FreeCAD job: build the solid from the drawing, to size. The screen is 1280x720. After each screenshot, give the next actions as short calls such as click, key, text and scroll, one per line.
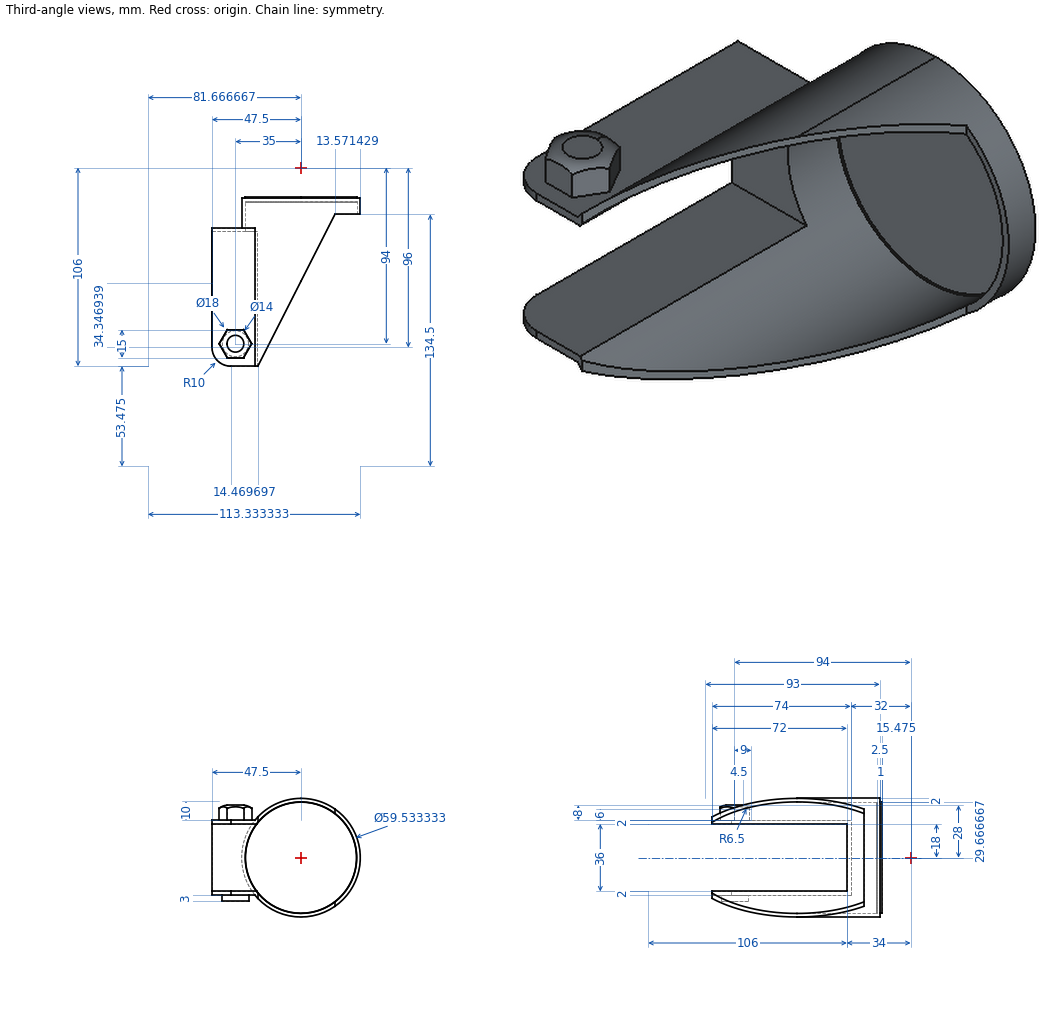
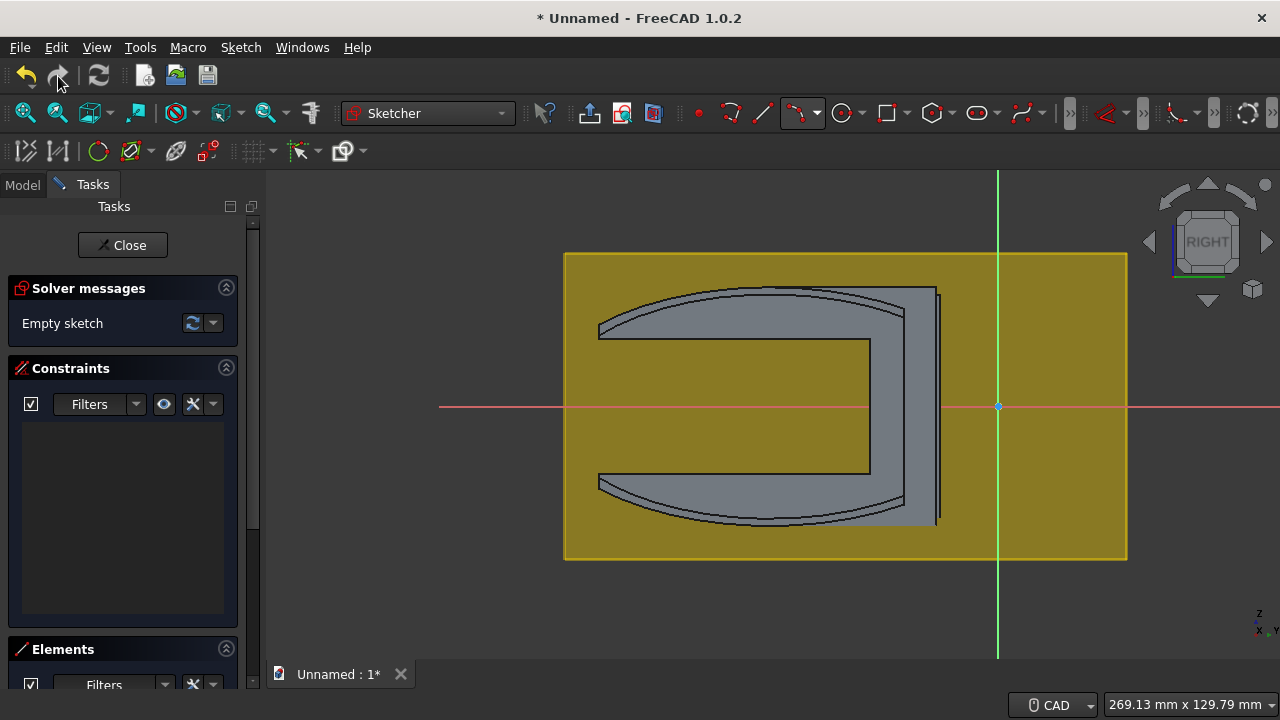
click(654, 114)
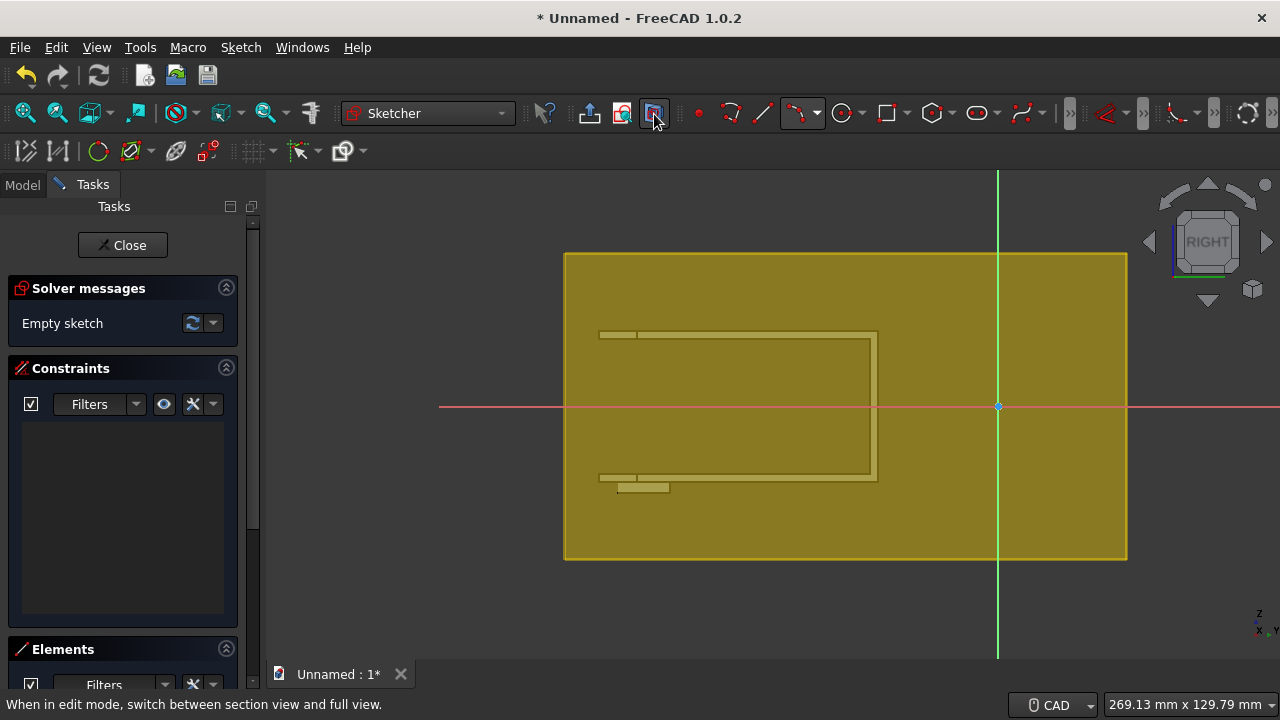
scroll(654, 294, up, 10)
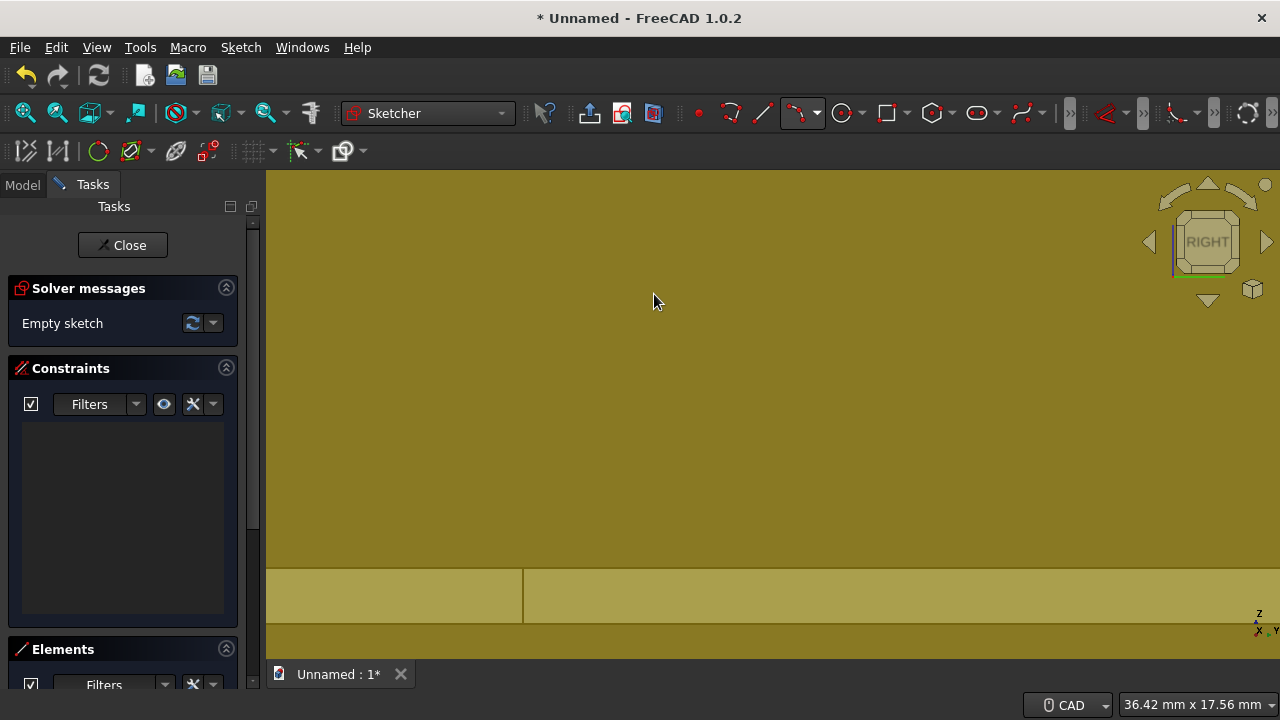
key(g)
key(m)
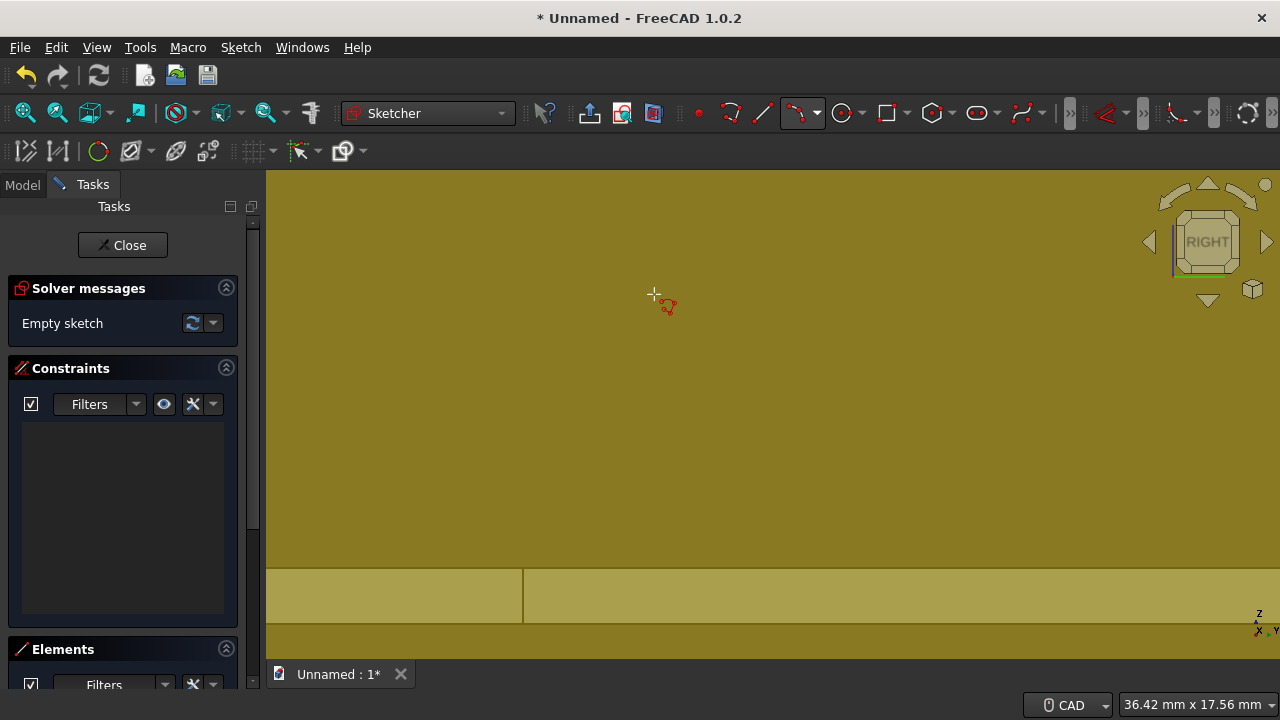
click(704, 345)
click(578, 345)
click(578, 568)
click(829, 568)
click(829, 401)
right_click(829, 401)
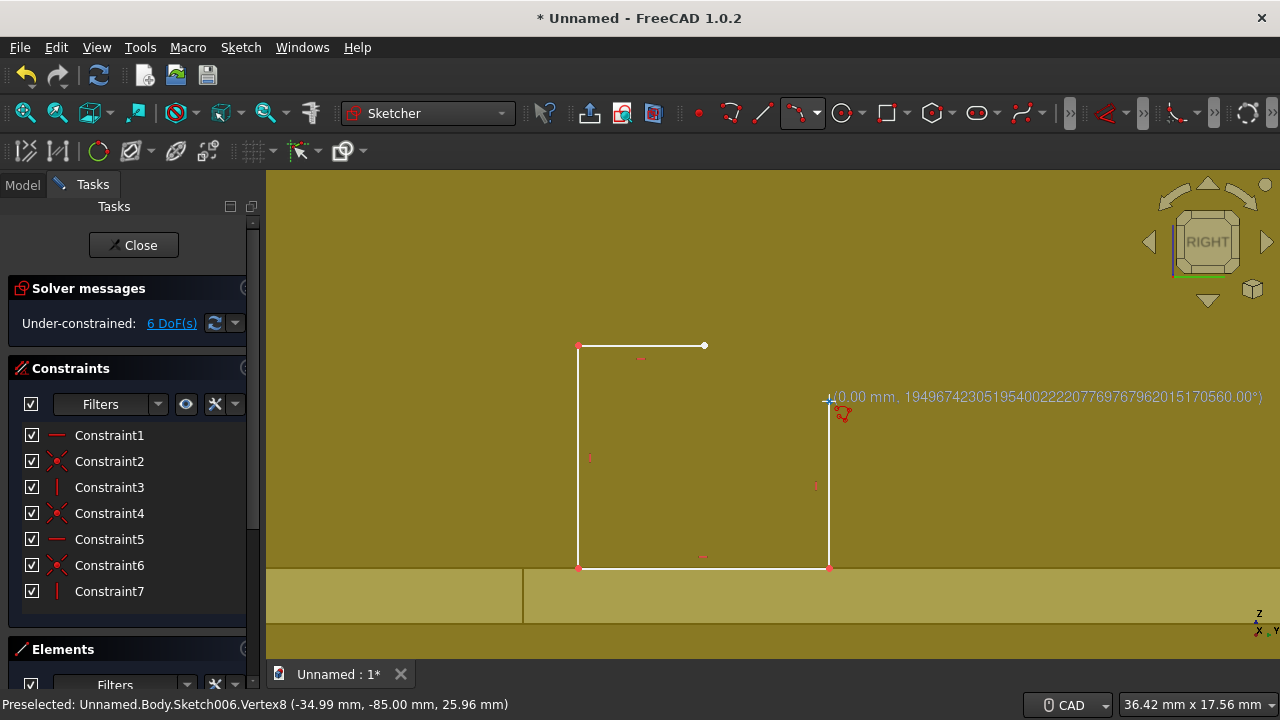
key(g)
key(3)
key(a)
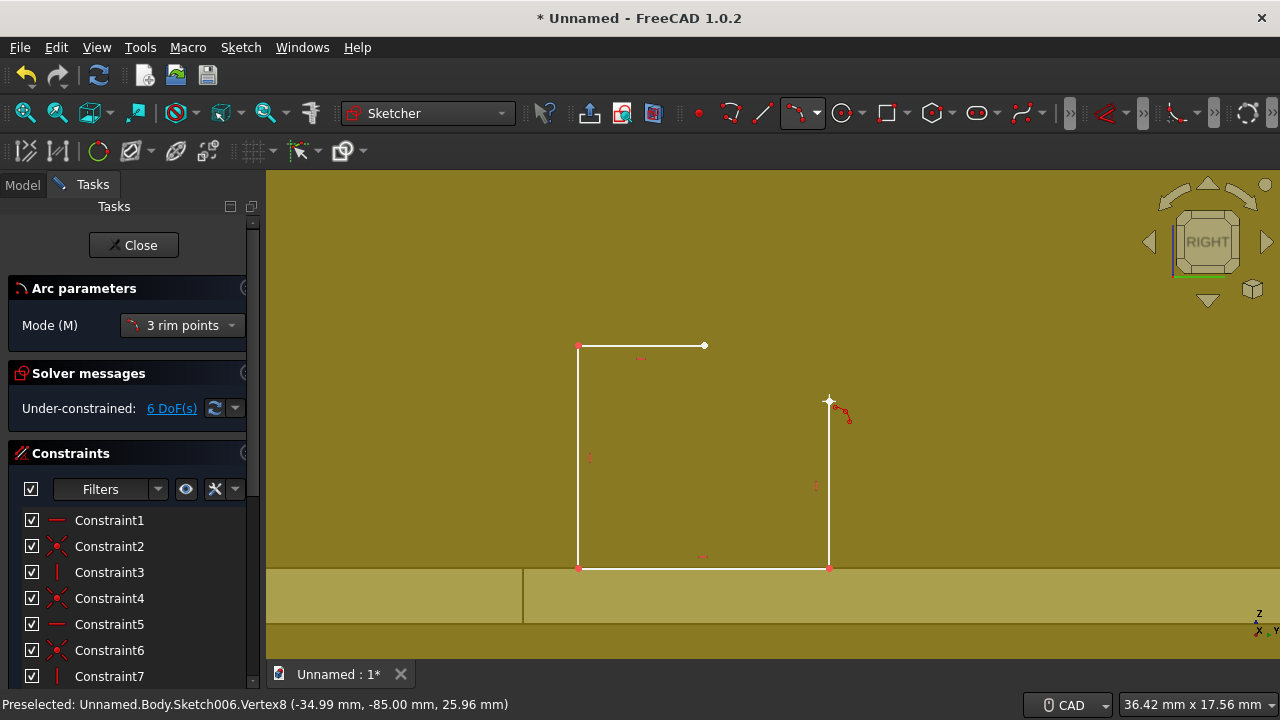
click(829, 402)
click(704, 346)
click(772, 361)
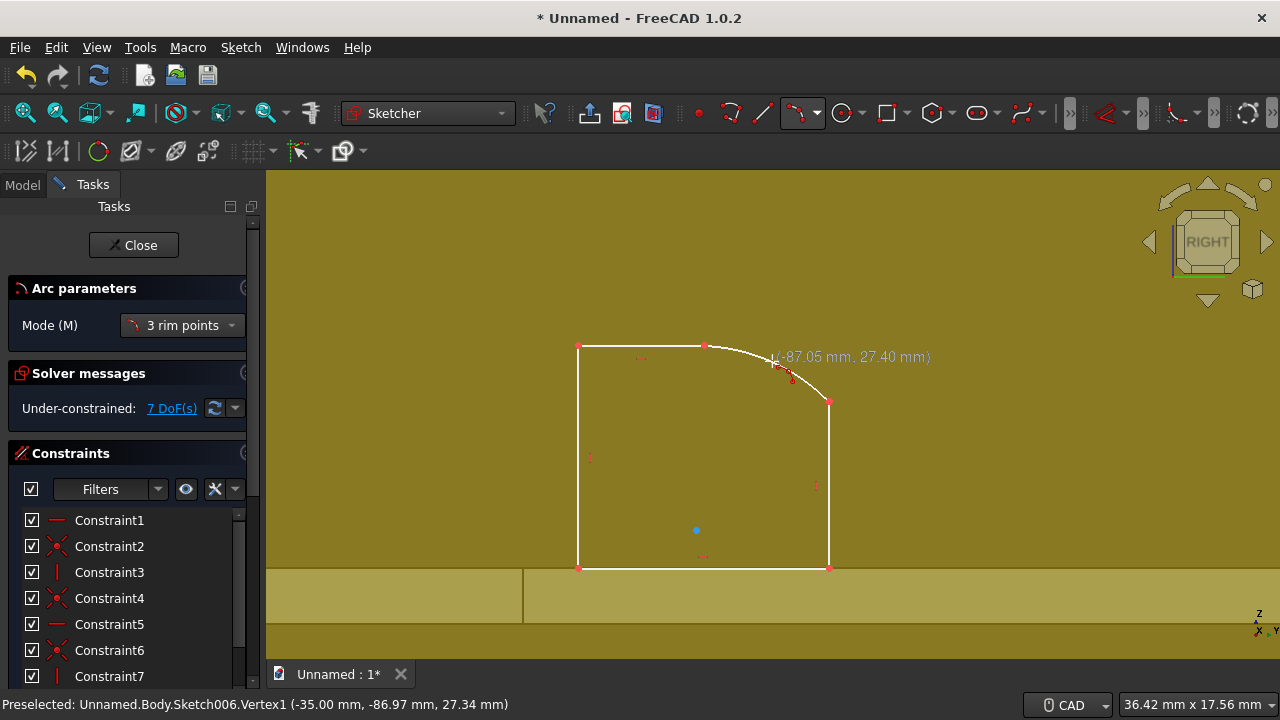
key(g)
key(l)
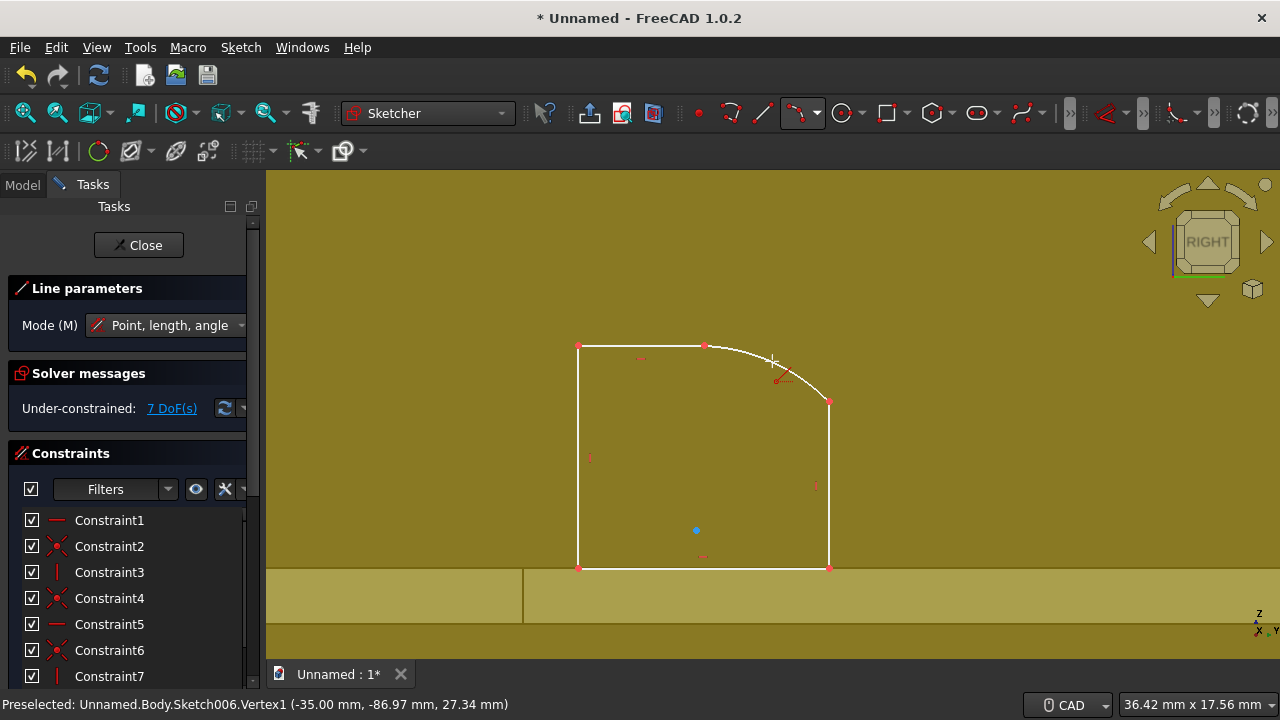
click(578, 323)
click(578, 256)
key(Escape)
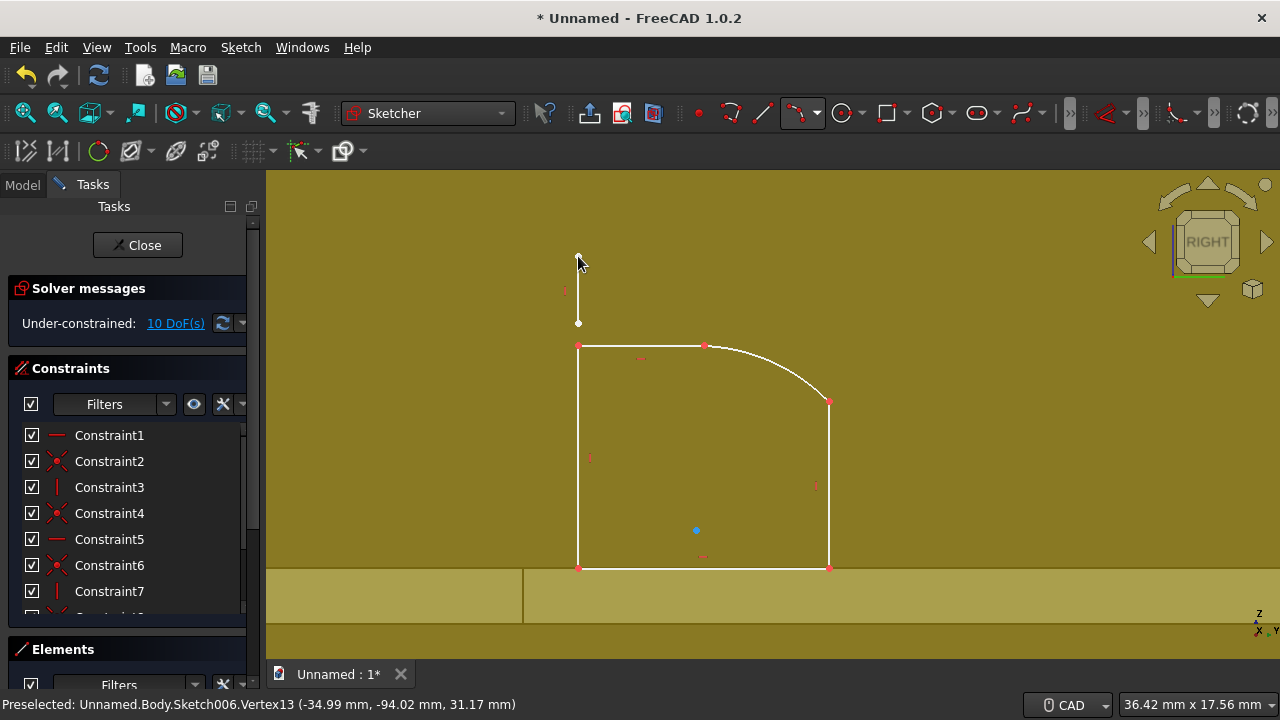
click(578, 304)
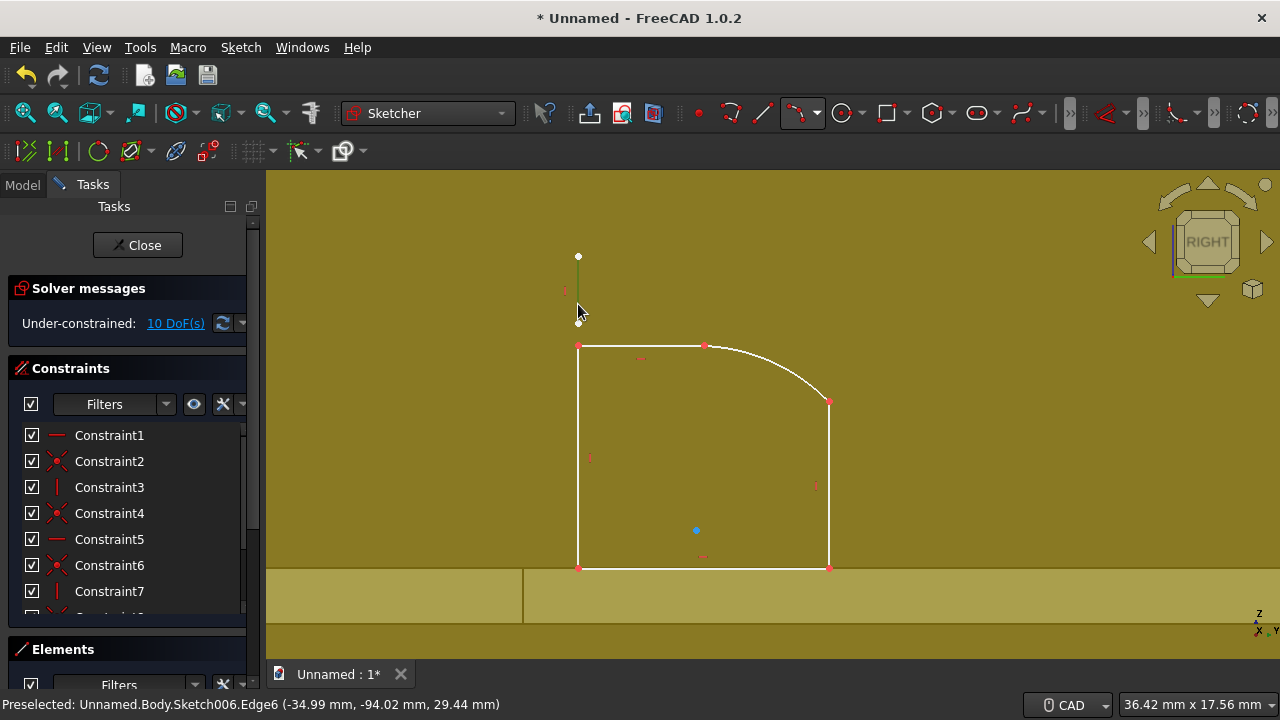
key(g)
key(n)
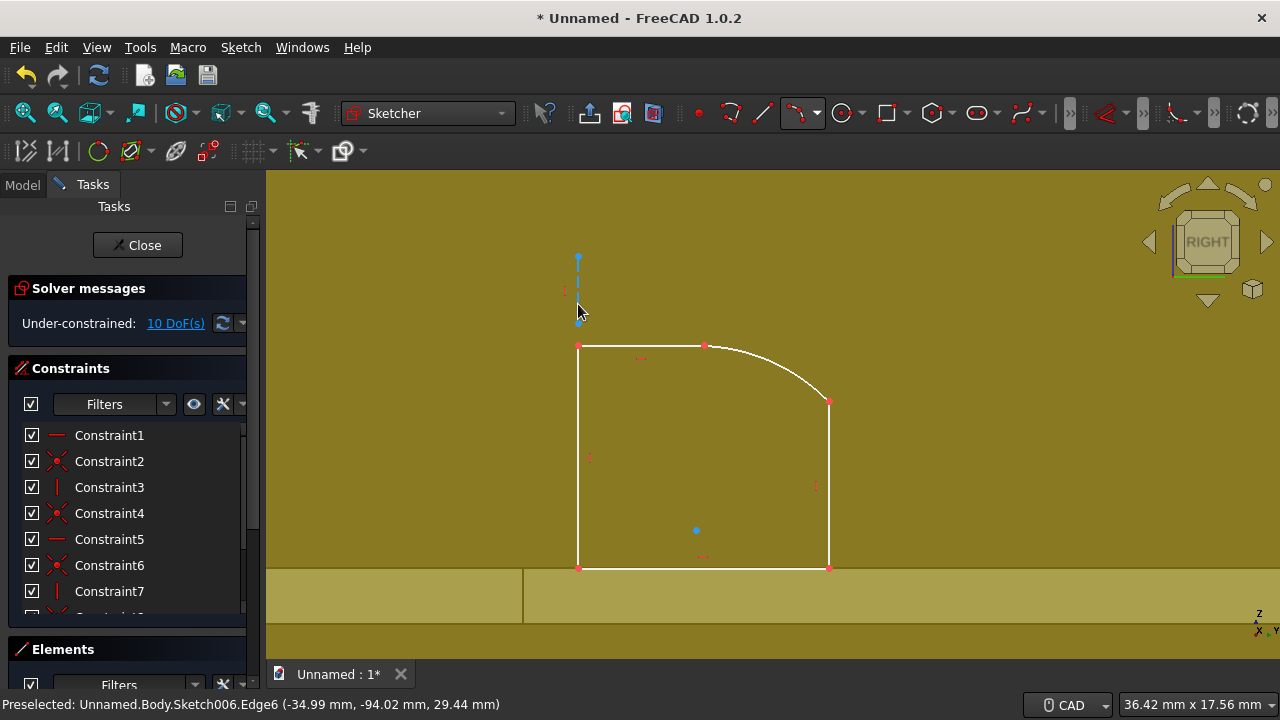
key(d)